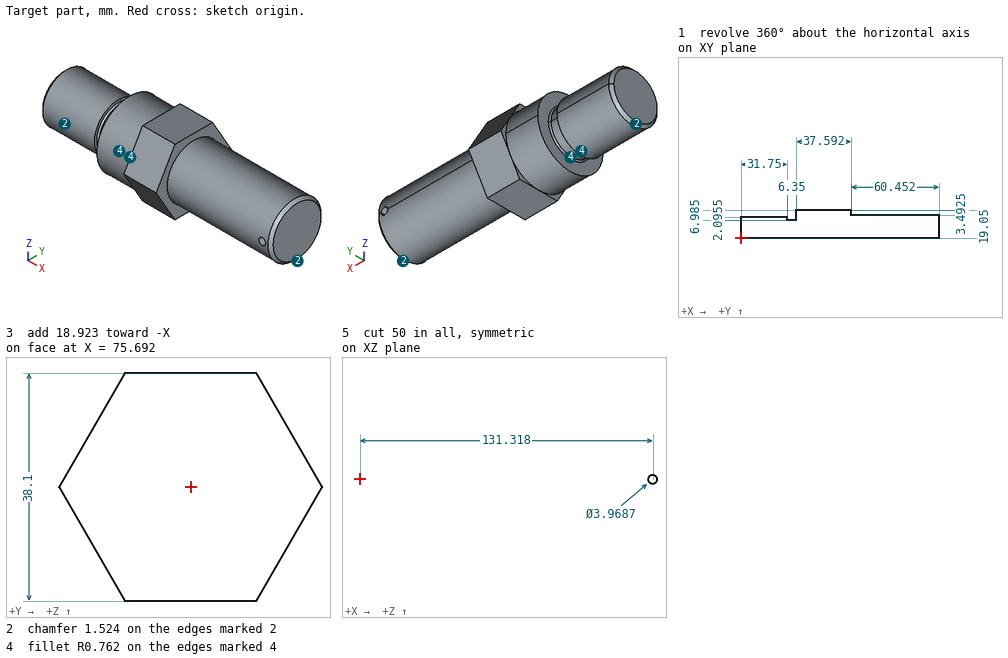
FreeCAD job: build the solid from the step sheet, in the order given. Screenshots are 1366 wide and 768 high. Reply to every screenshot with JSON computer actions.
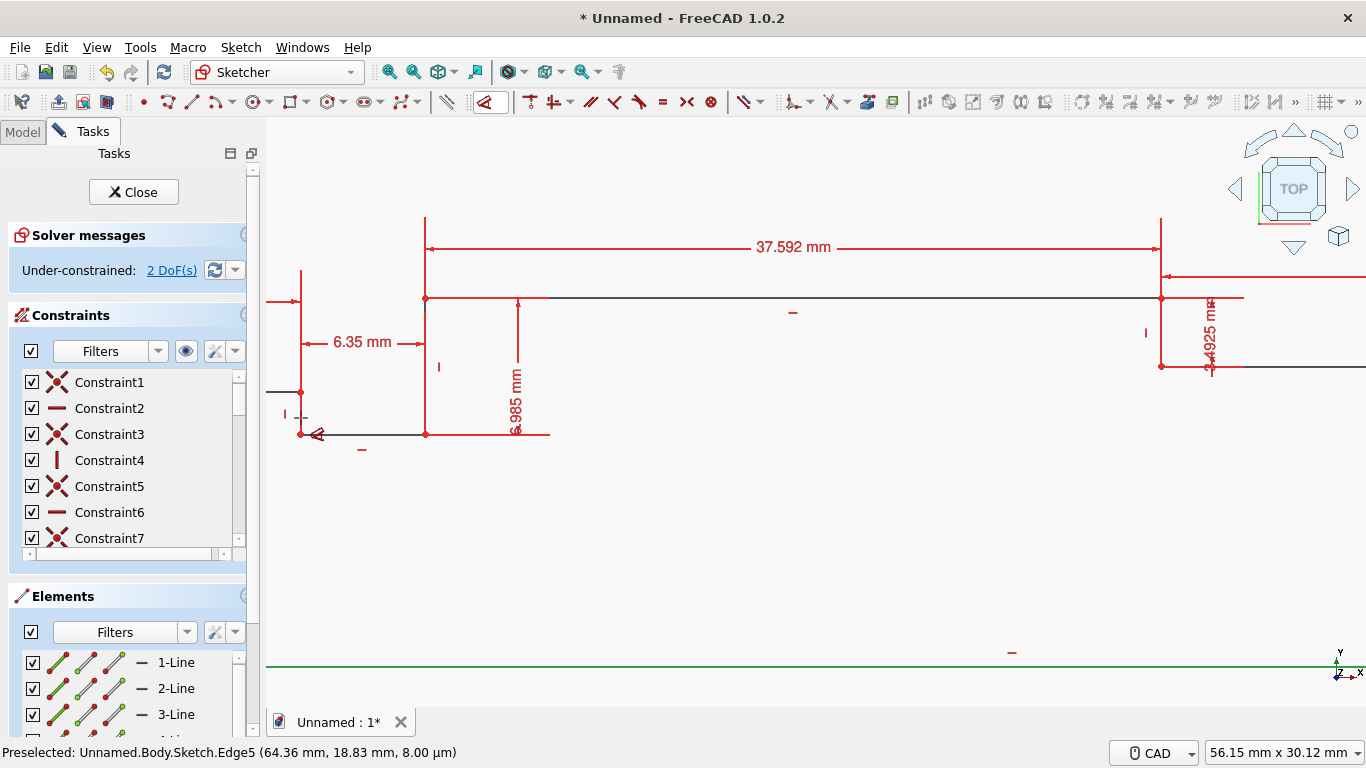
{"action": "left_click", "coordinate": [301, 418]}
{"action": "left_click", "coordinate": [335, 414]}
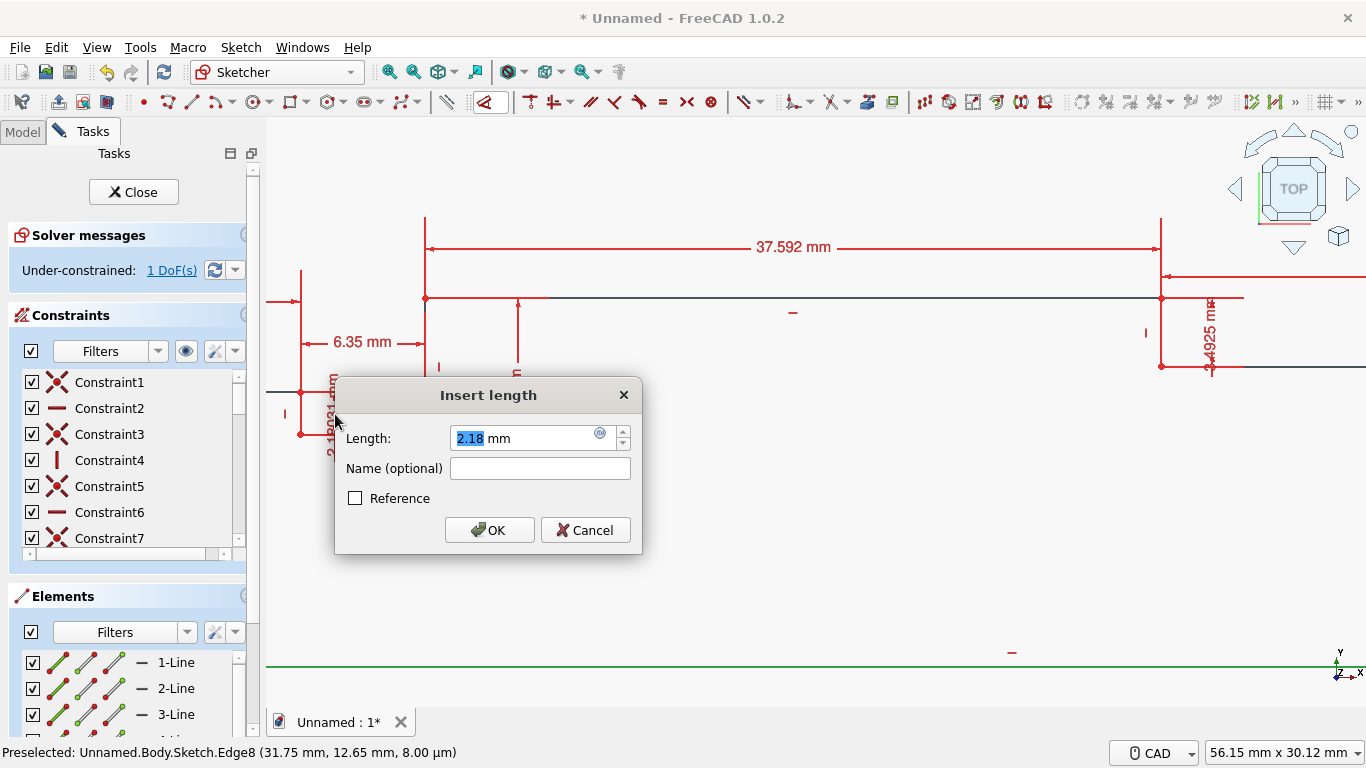
{"action": "type", "text": "2.0955"}
{"action": "key", "text": "Return"}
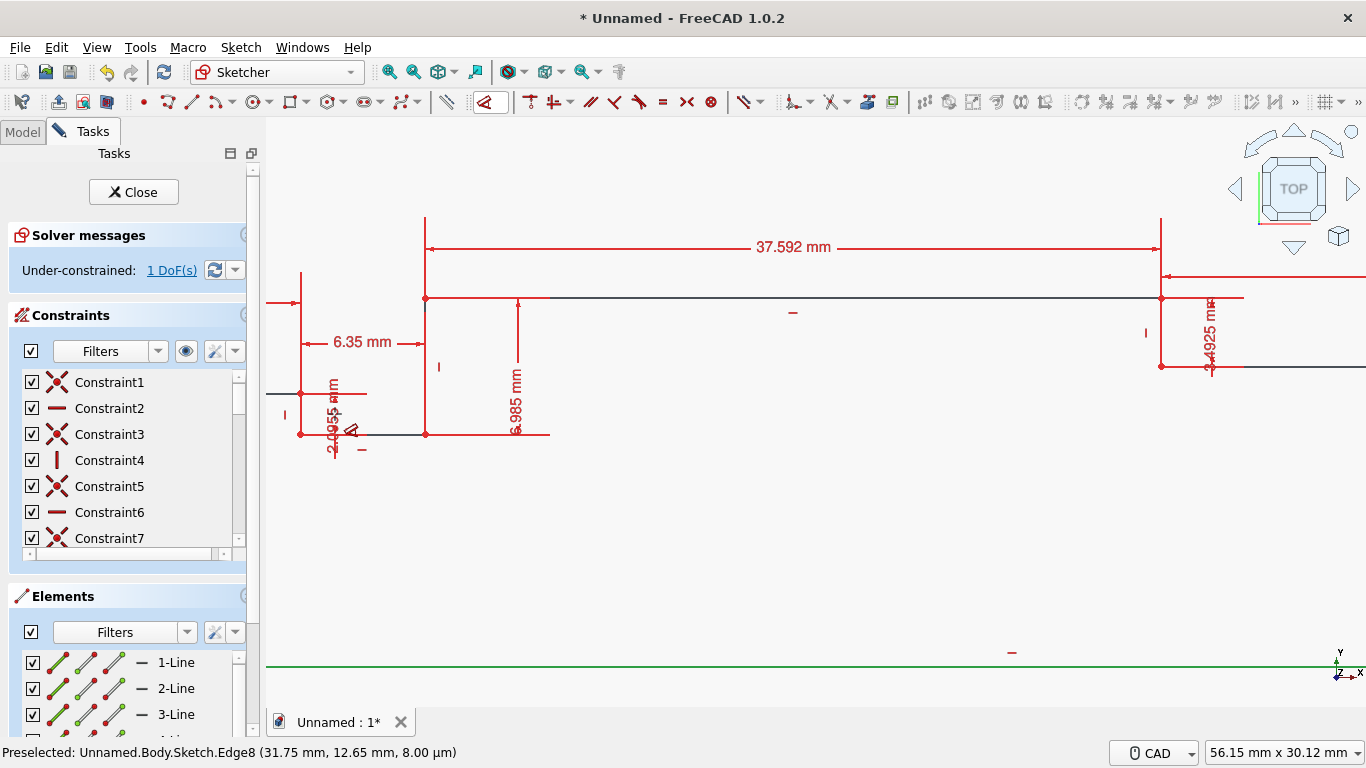
{"action": "scroll", "coordinate": [661, 390], "scroll_direction": "down", "scroll_amount": 7}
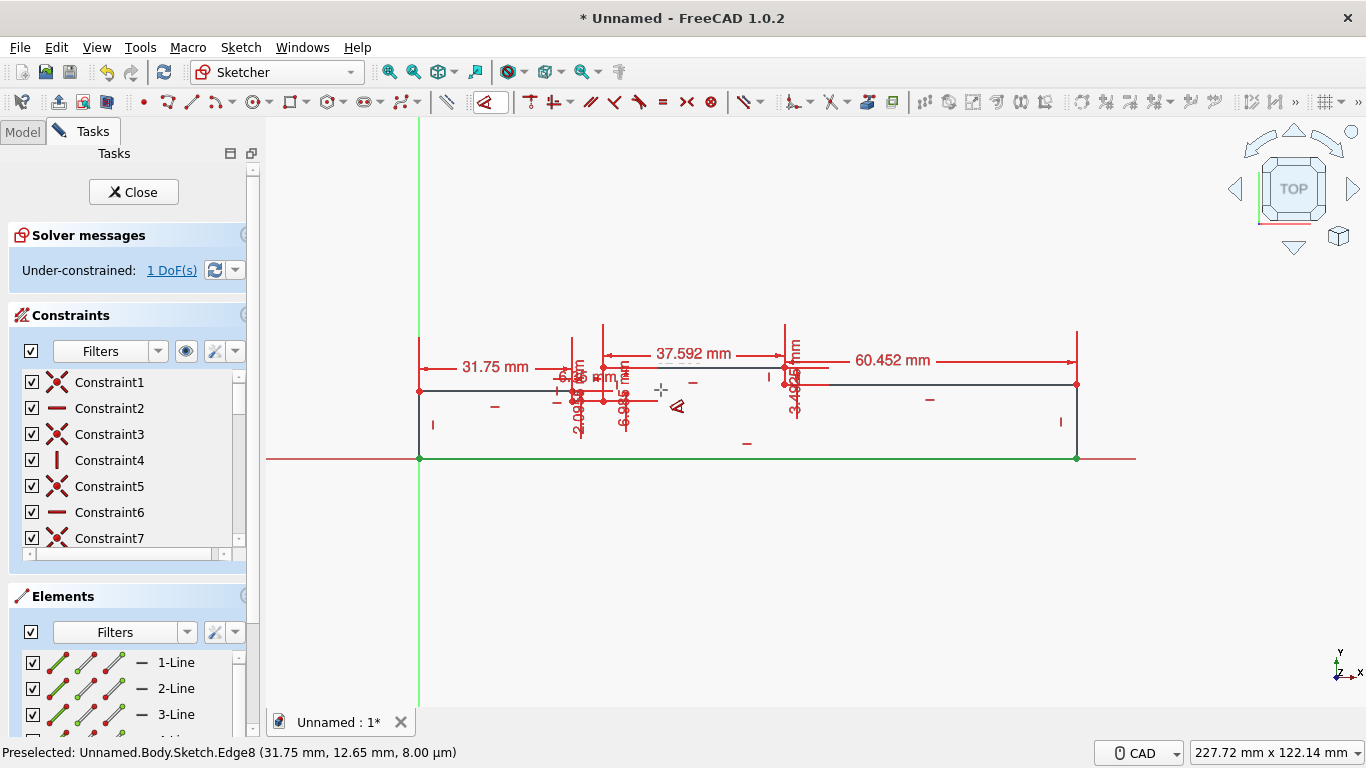
{"action": "left_click", "coordinate": [785, 368]}
{"action": "left_click", "coordinate": [385, 413]}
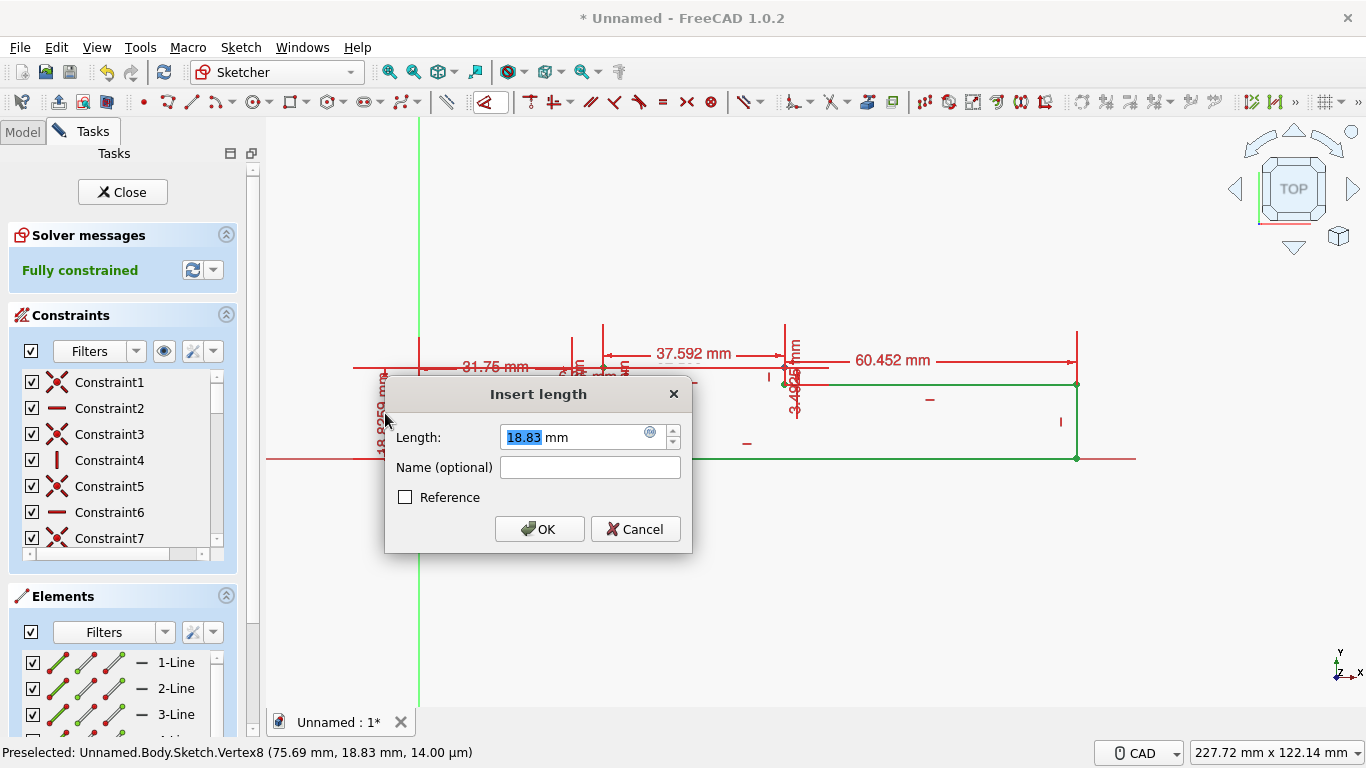
{"action": "type", "text": "19.05"}
{"action": "key", "text": "Return"}
{"action": "key", "text": "Escape"}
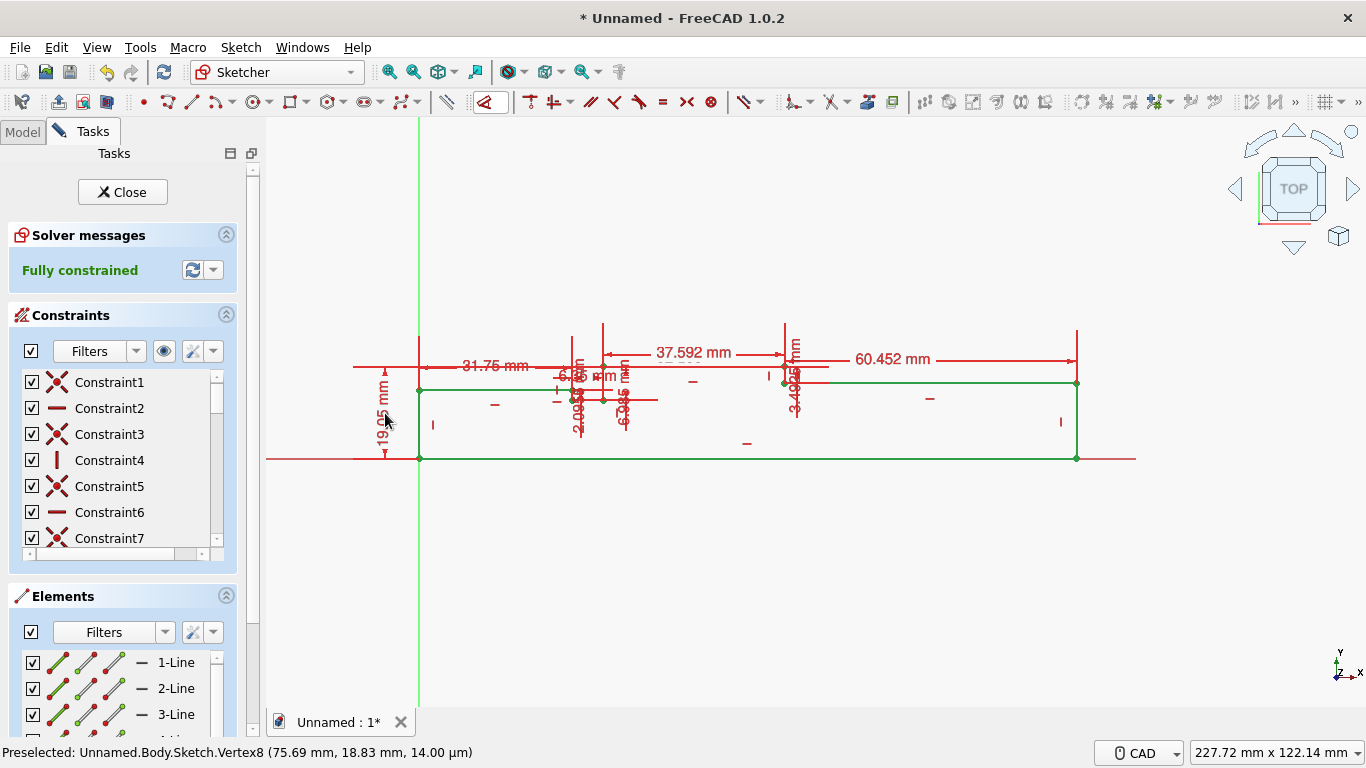
{"action": "left_click", "coordinate": [123, 192]}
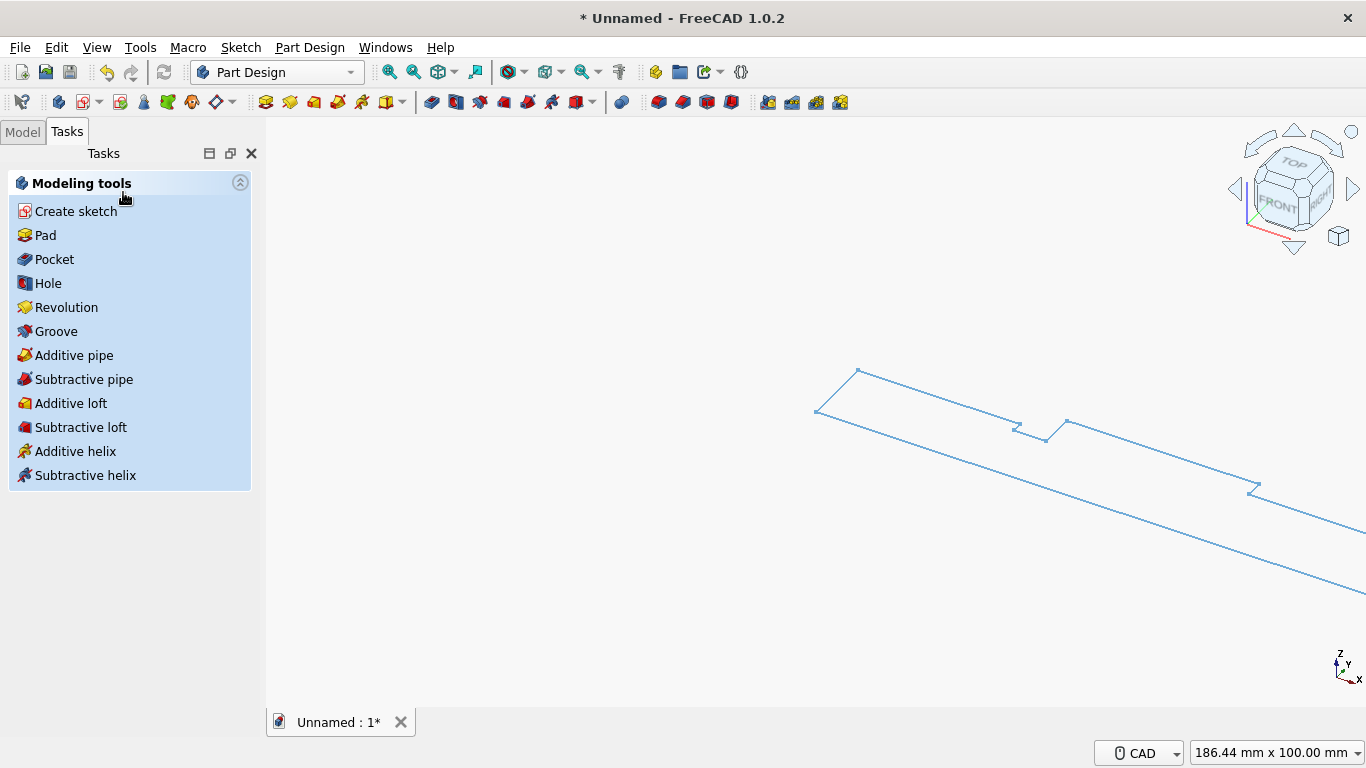
{"action": "left_click", "coordinate": [290, 102]}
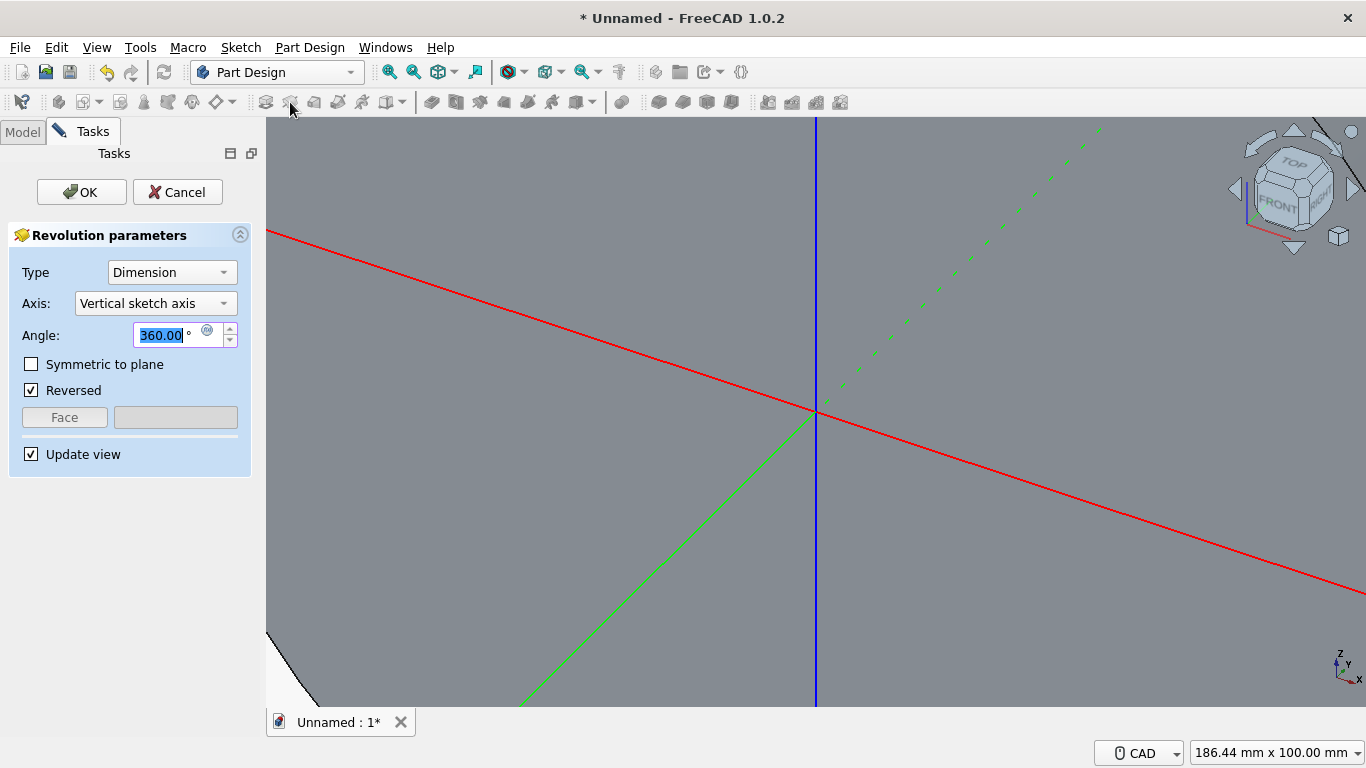
{"action": "left_click", "coordinate": [156, 304]}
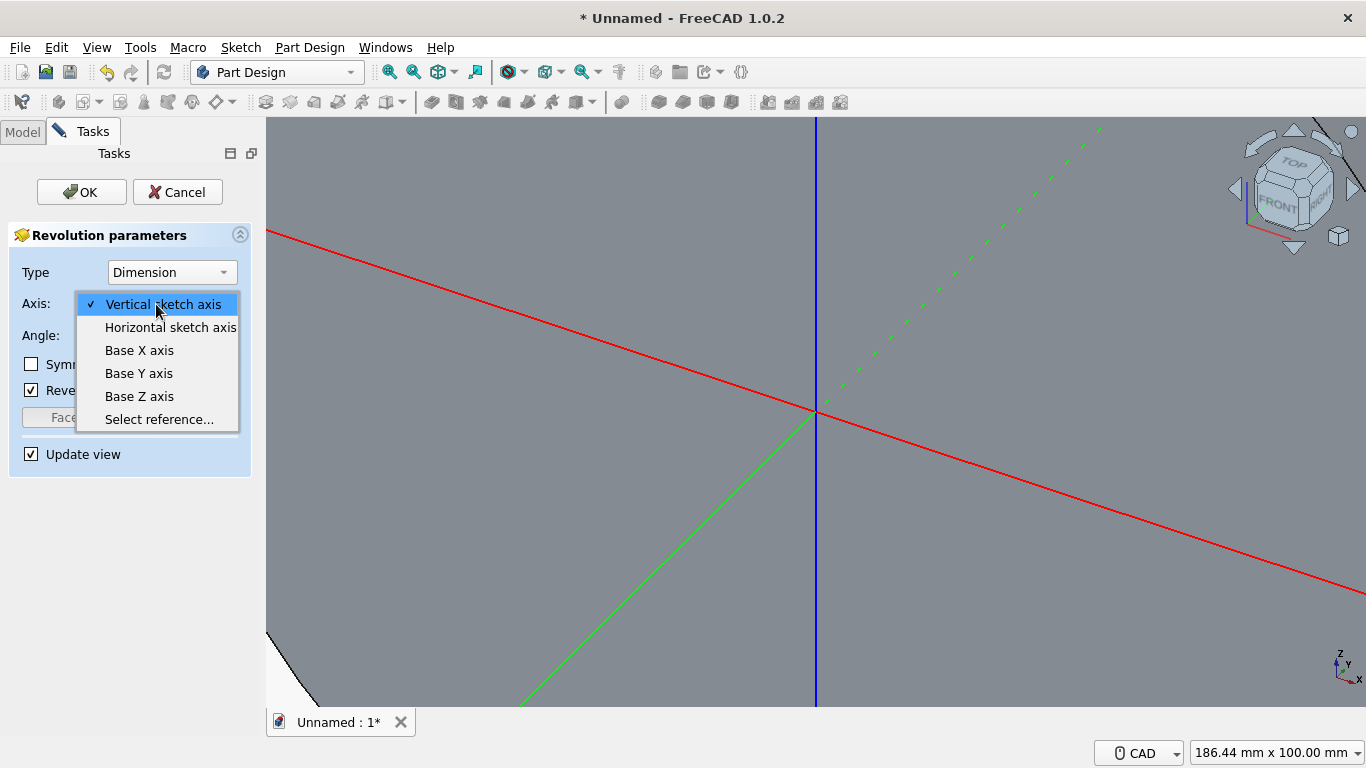
{"action": "left_click", "coordinate": [156, 328]}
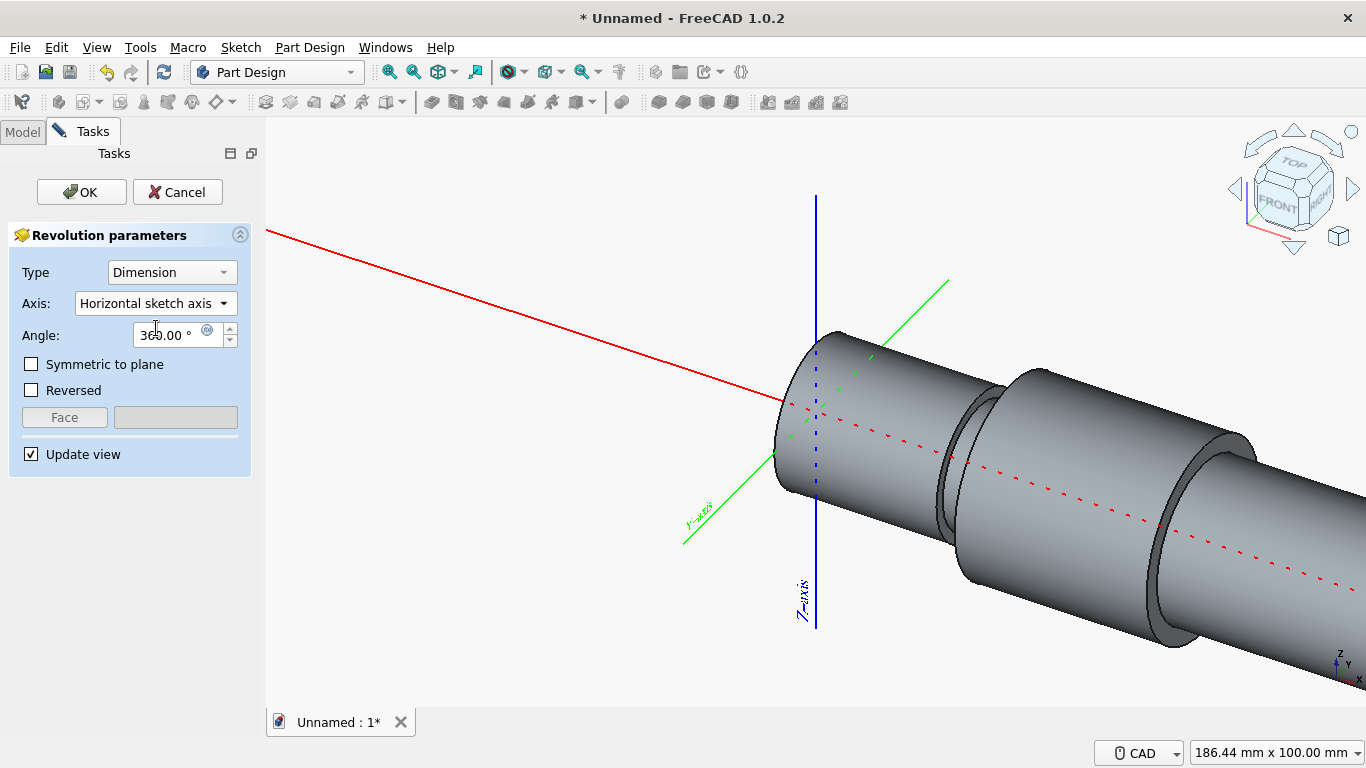
{"action": "left_click", "coordinate": [82, 192]}